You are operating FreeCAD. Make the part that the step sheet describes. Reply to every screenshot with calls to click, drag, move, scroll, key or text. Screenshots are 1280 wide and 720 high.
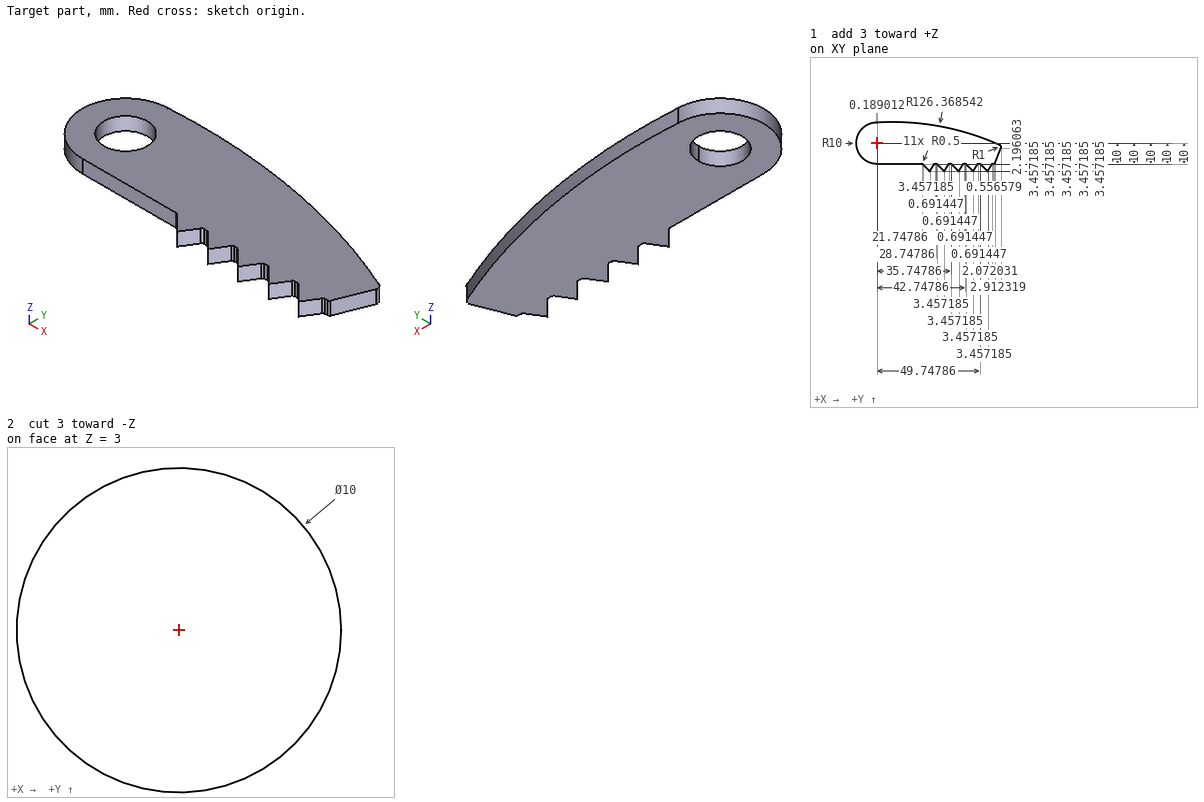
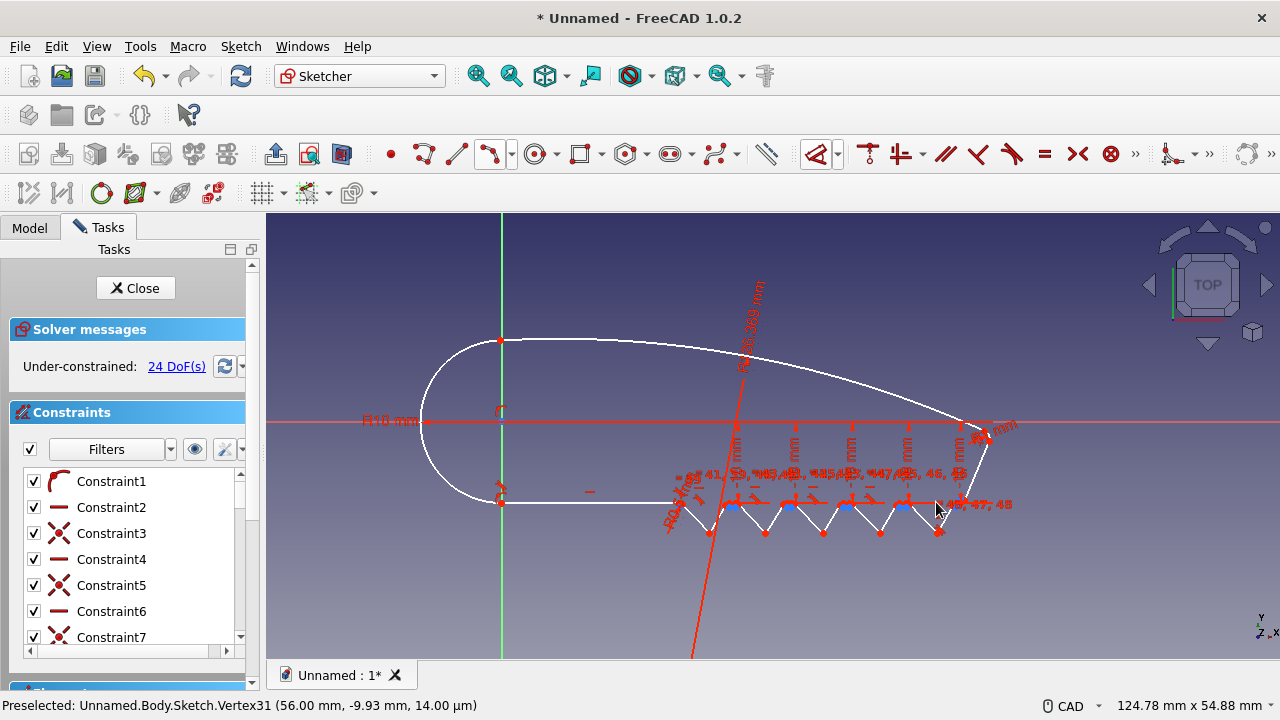
click(555, 503)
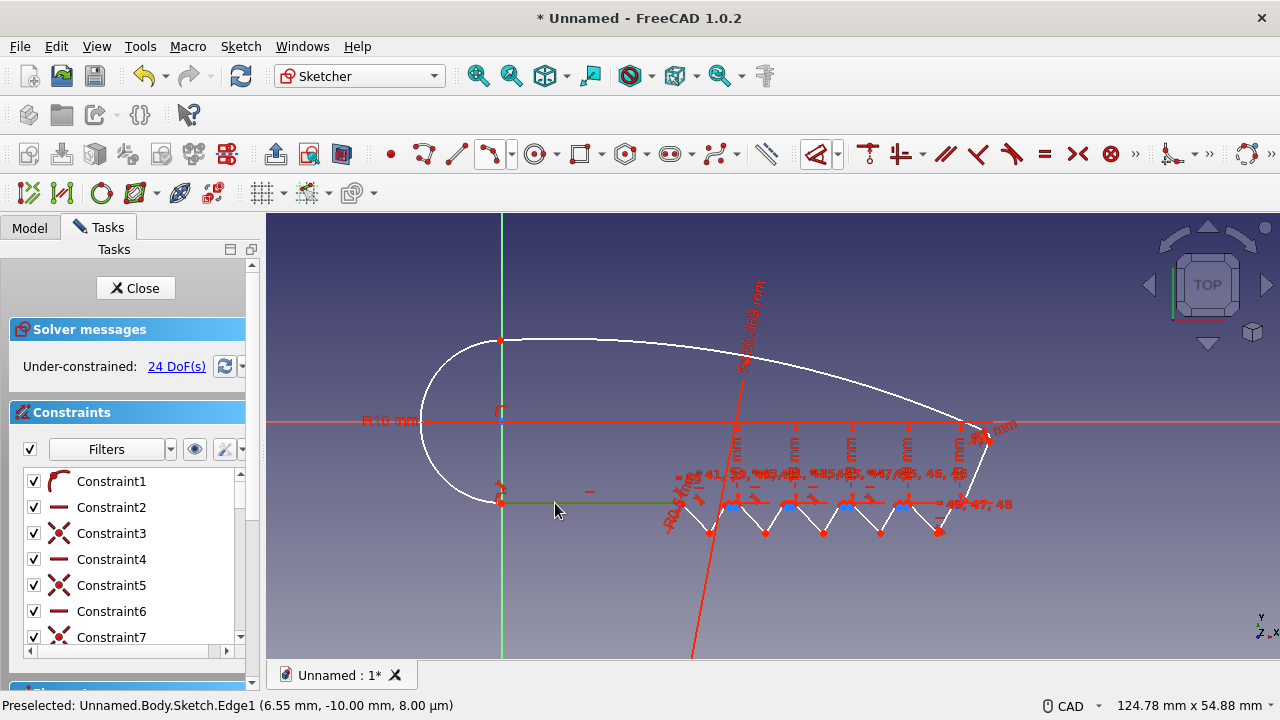
click(838, 154)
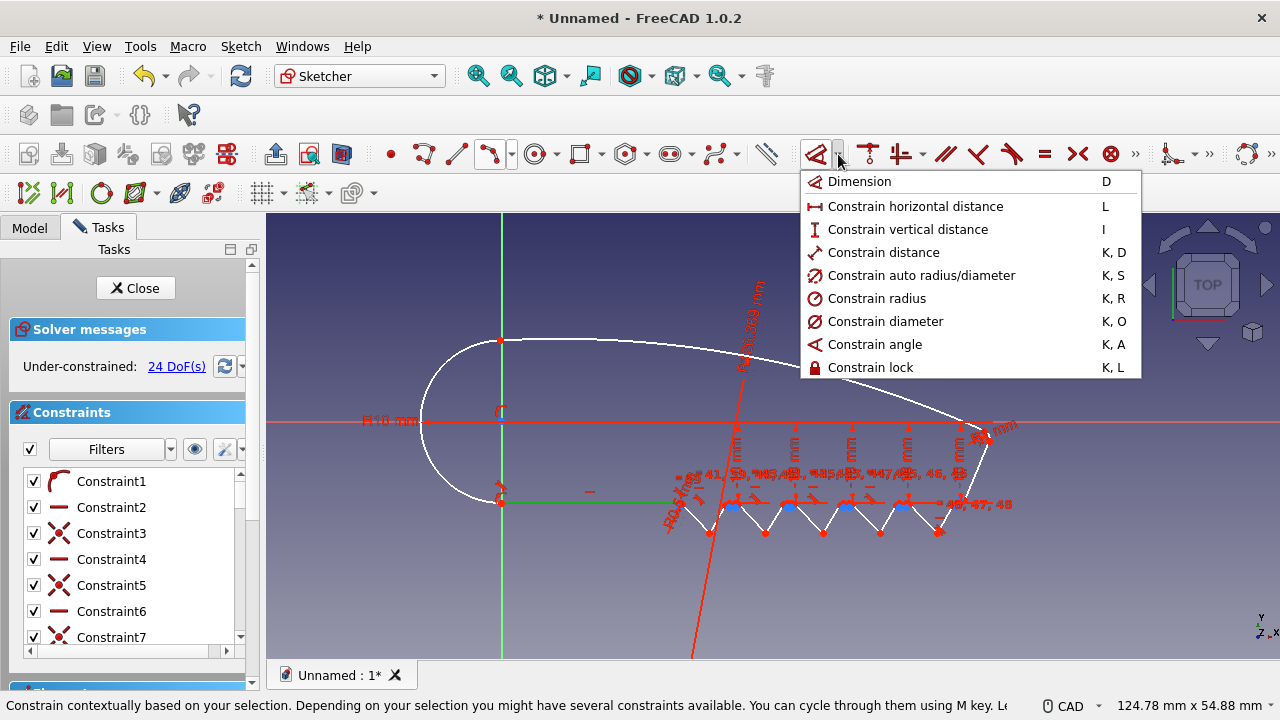
click(971, 206)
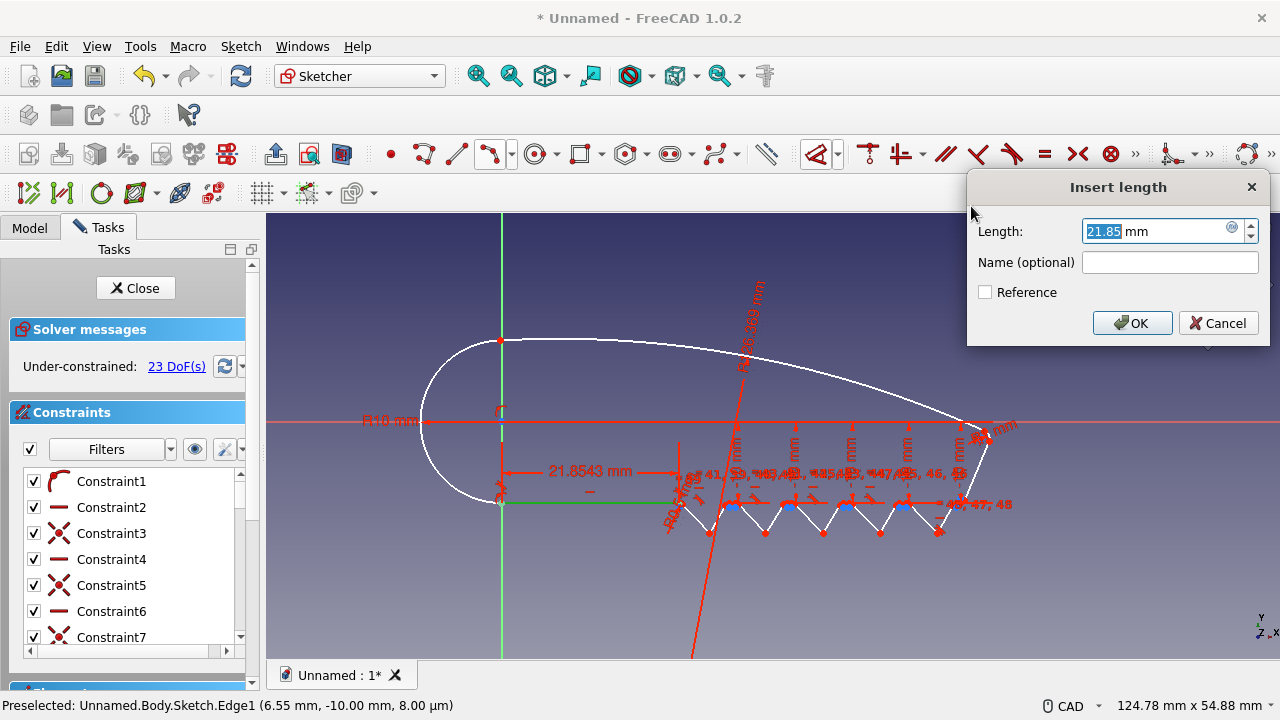
text(21.74786)
key(Return)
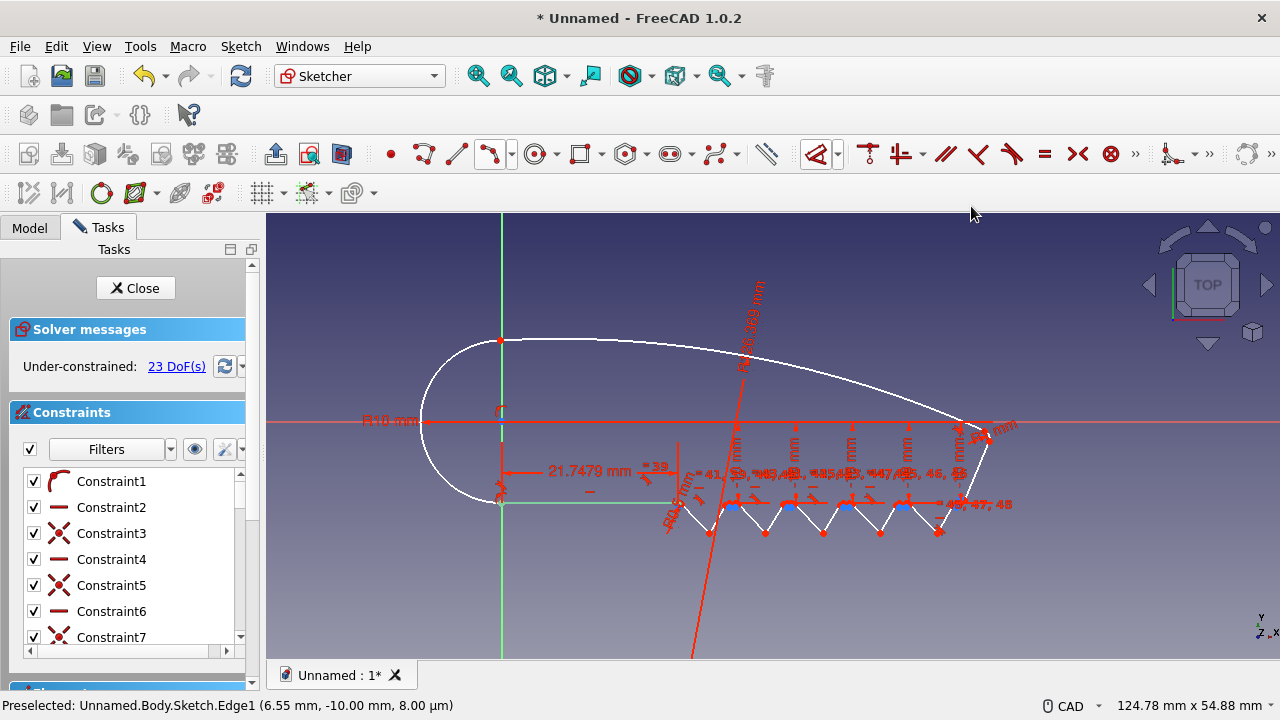
scroll(733, 503, up, 10)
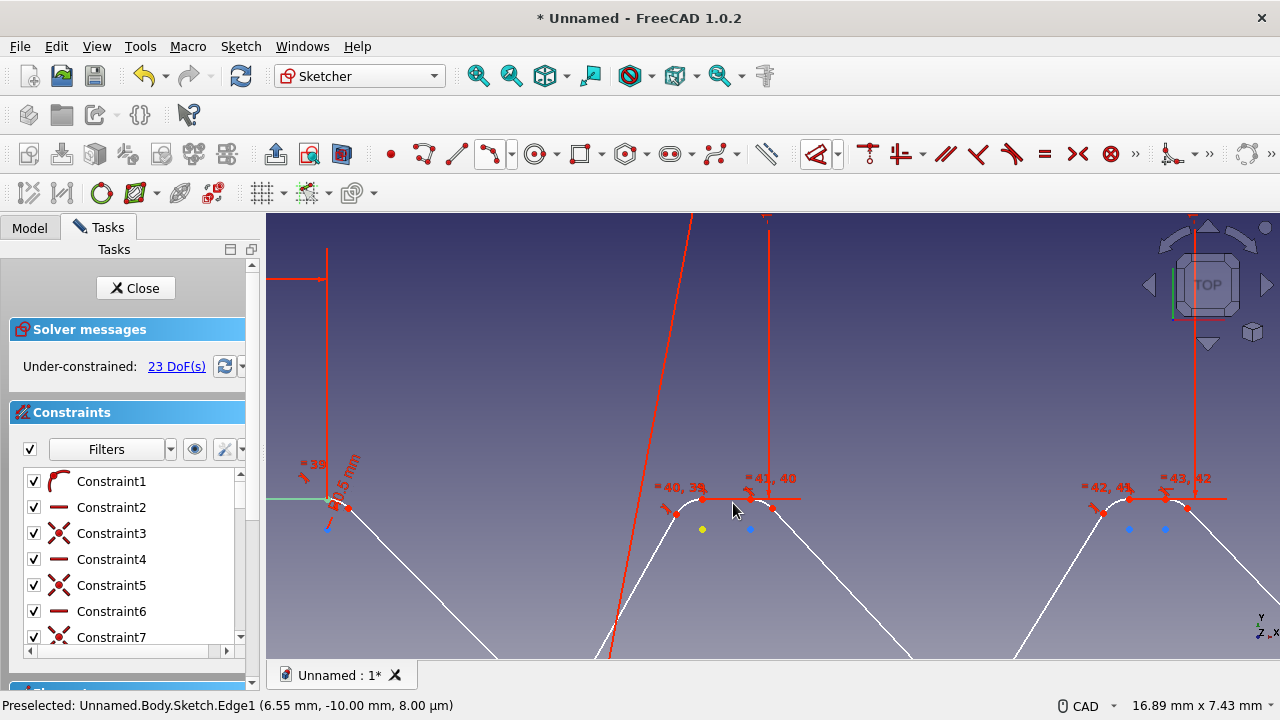
click(726, 499)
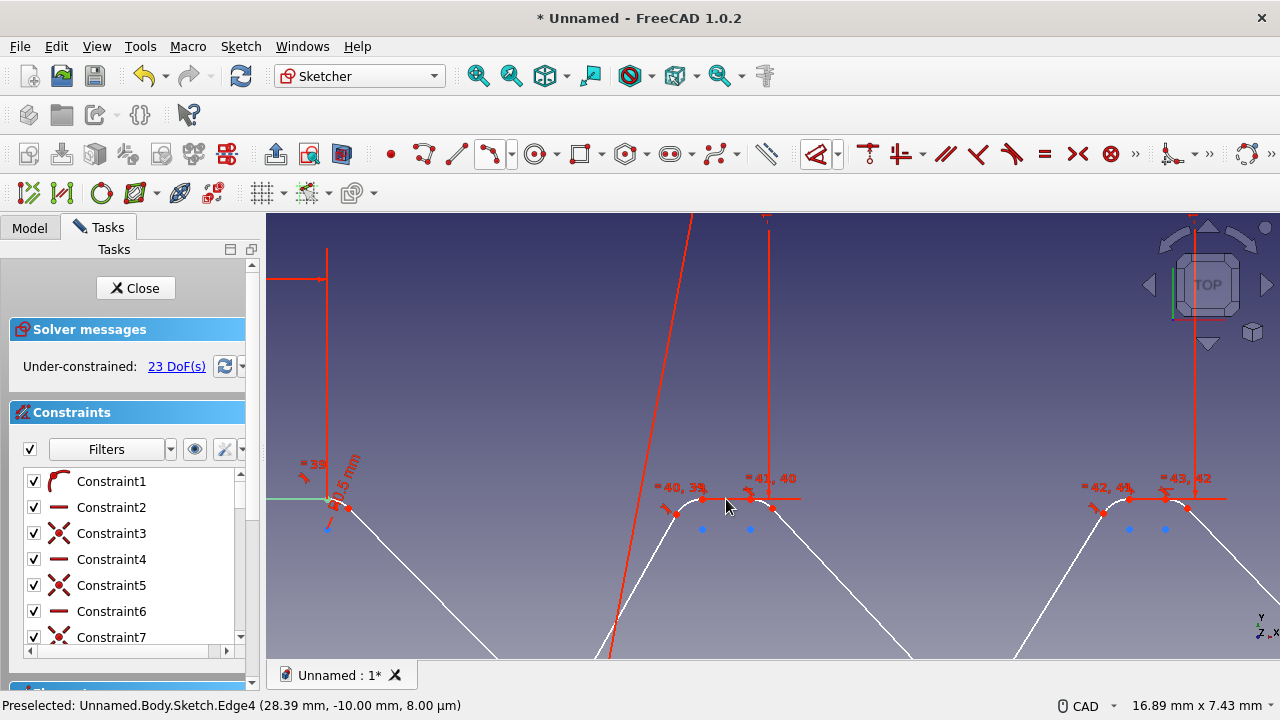
key(l)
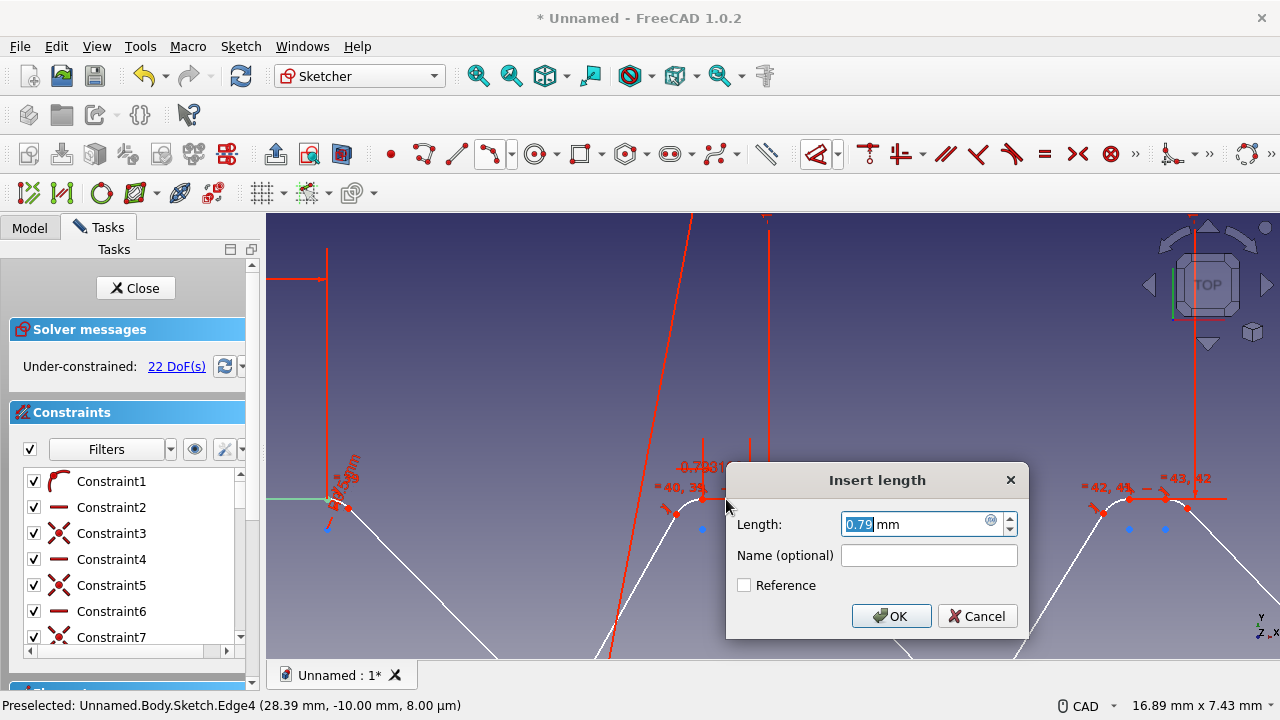
text(0.691447)
key(Return)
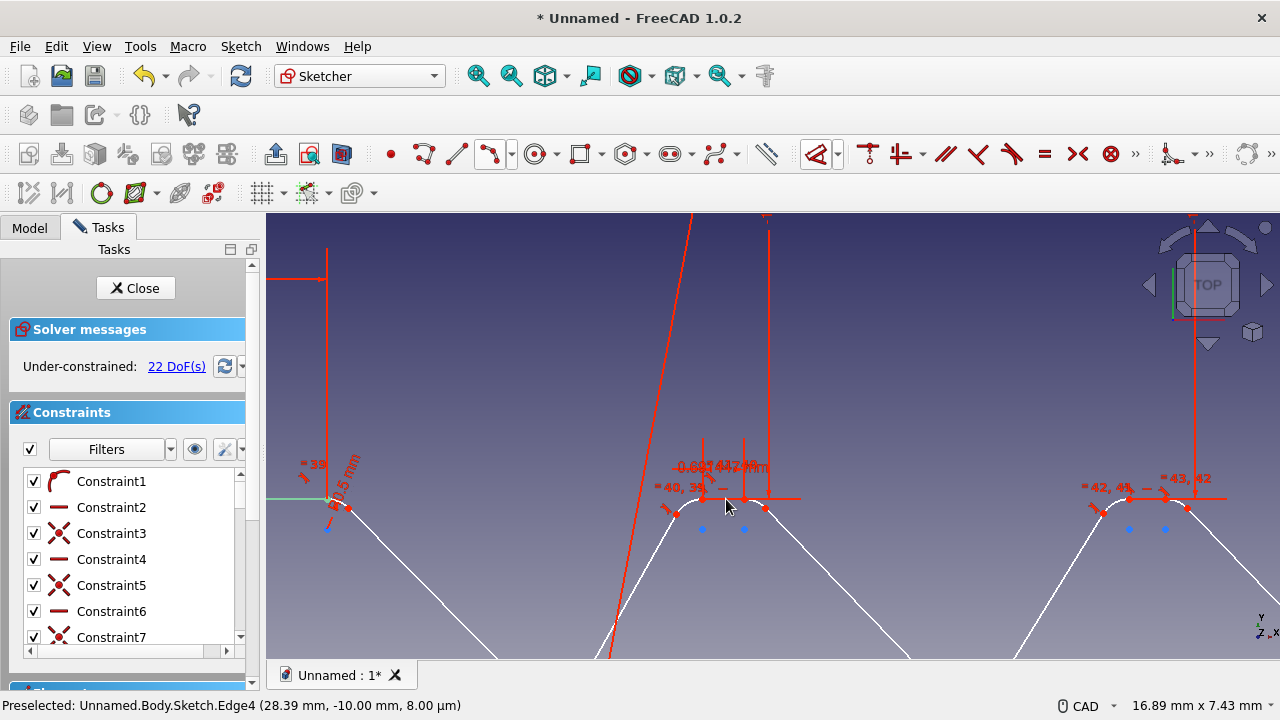
scroll(733, 503, down, 10)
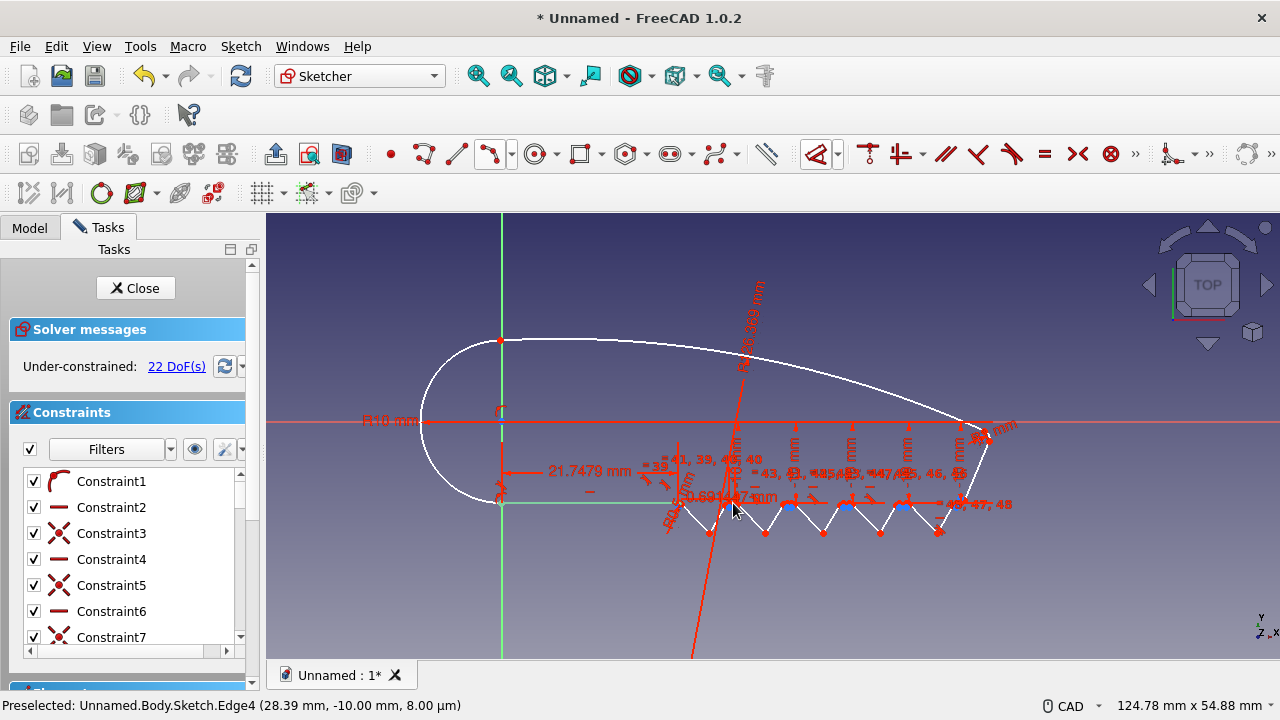
scroll(789, 503, up, 12)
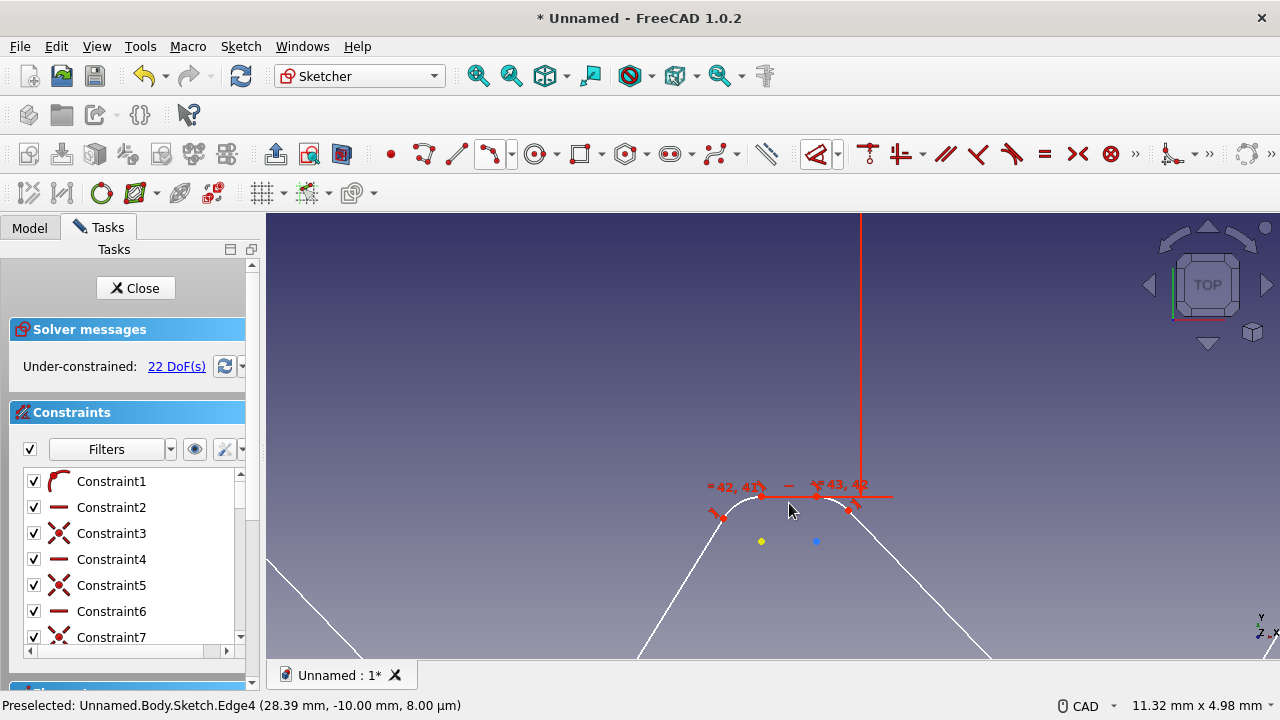
click(778, 497)